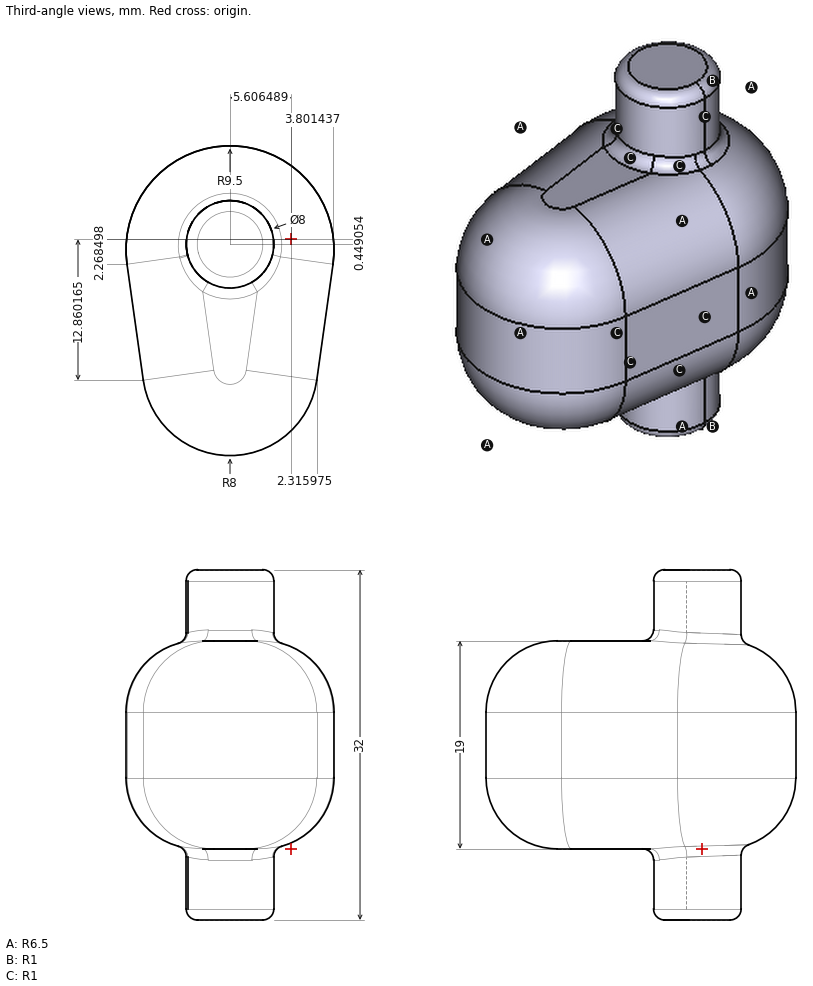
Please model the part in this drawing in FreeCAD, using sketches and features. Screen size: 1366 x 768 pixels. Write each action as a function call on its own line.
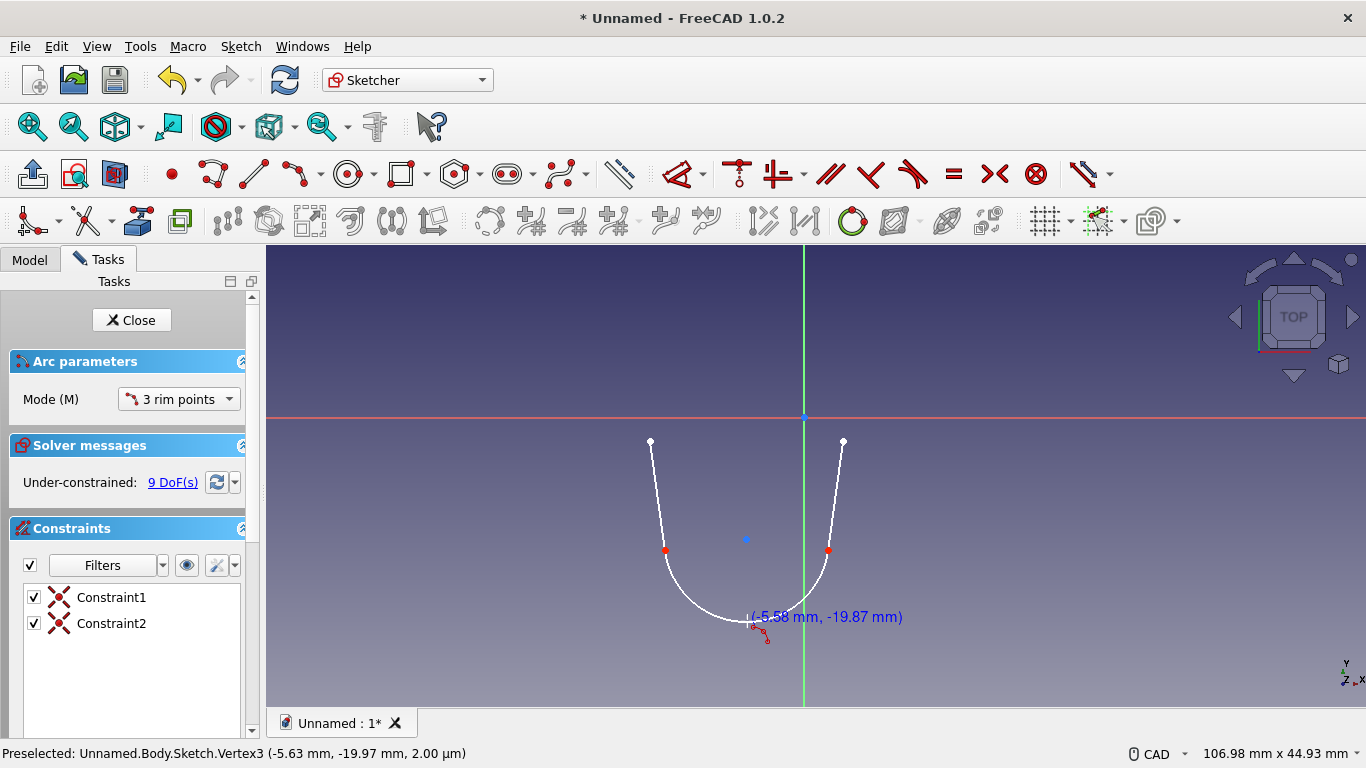
click(843, 442)
click(650, 442)
click(747, 330)
key(Escape)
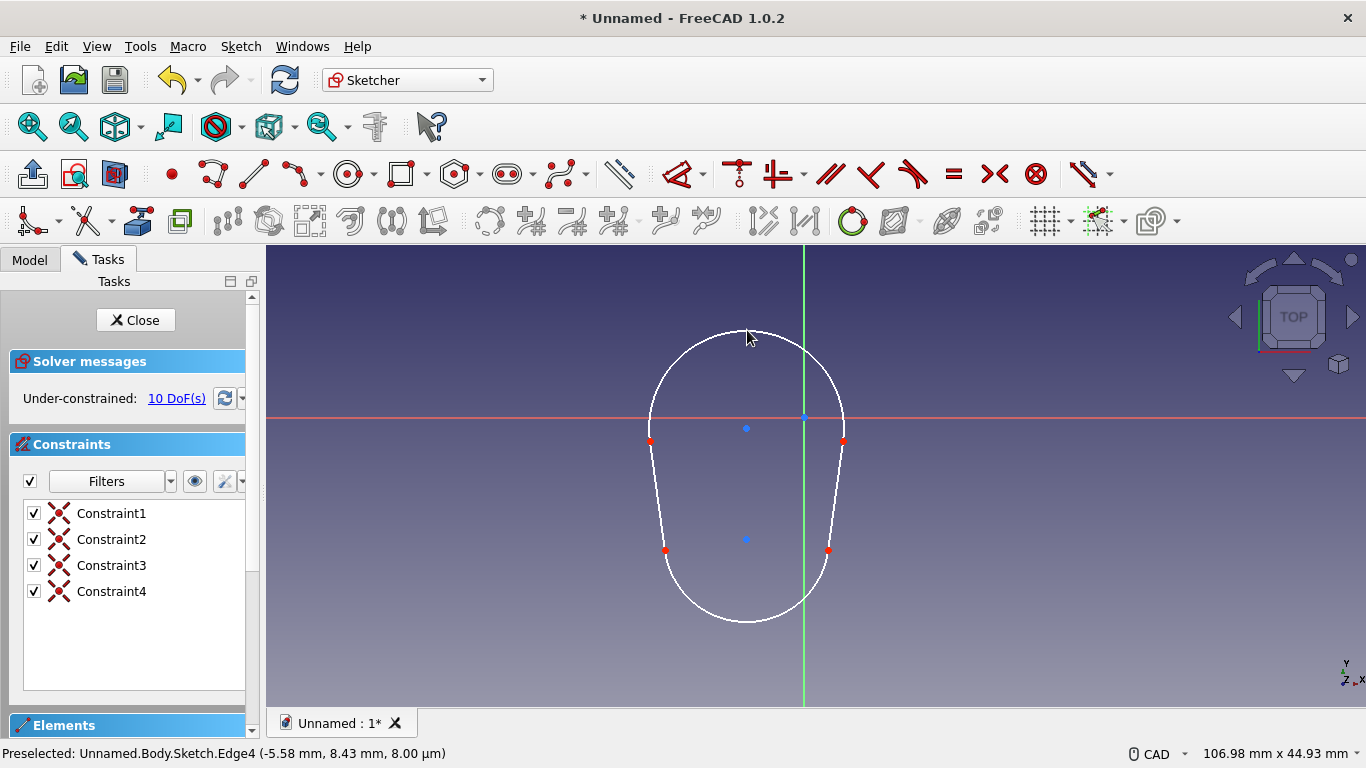
click(654, 475)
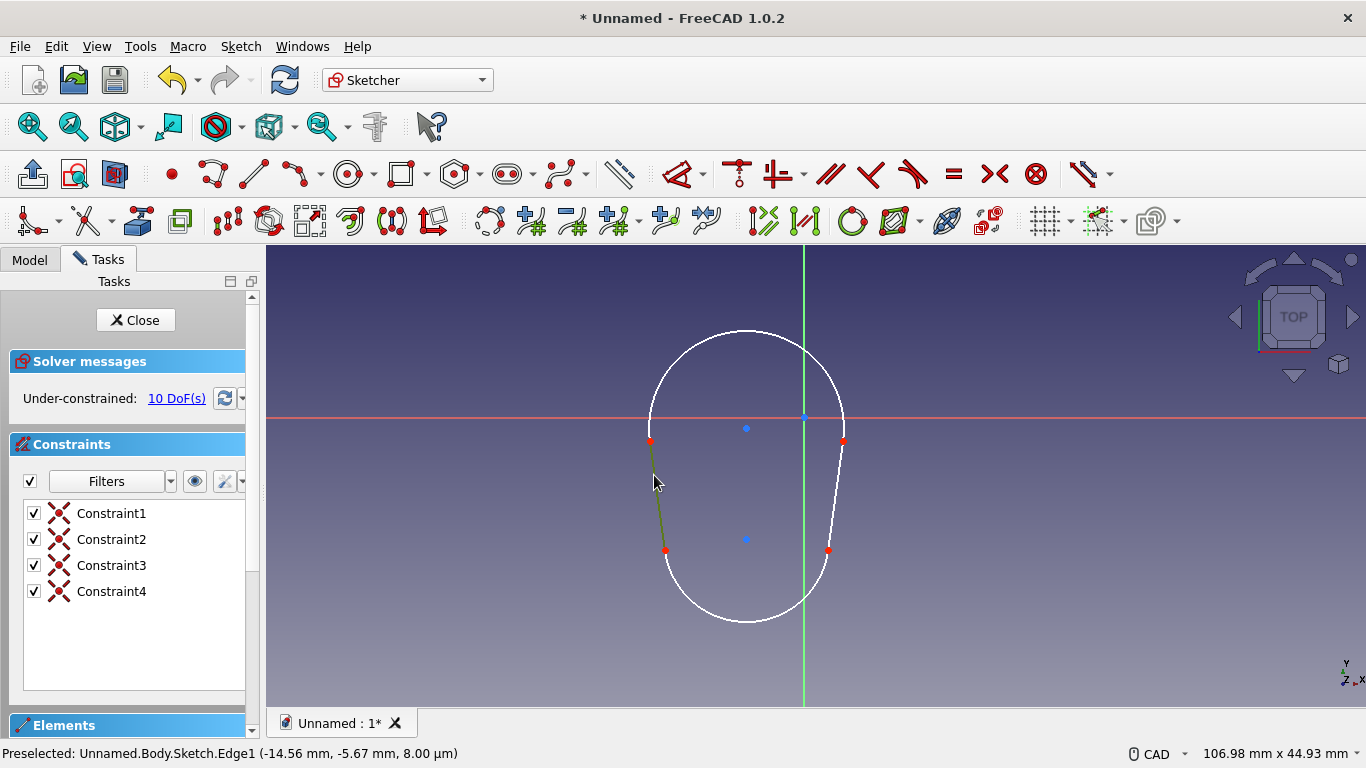
click(702, 609)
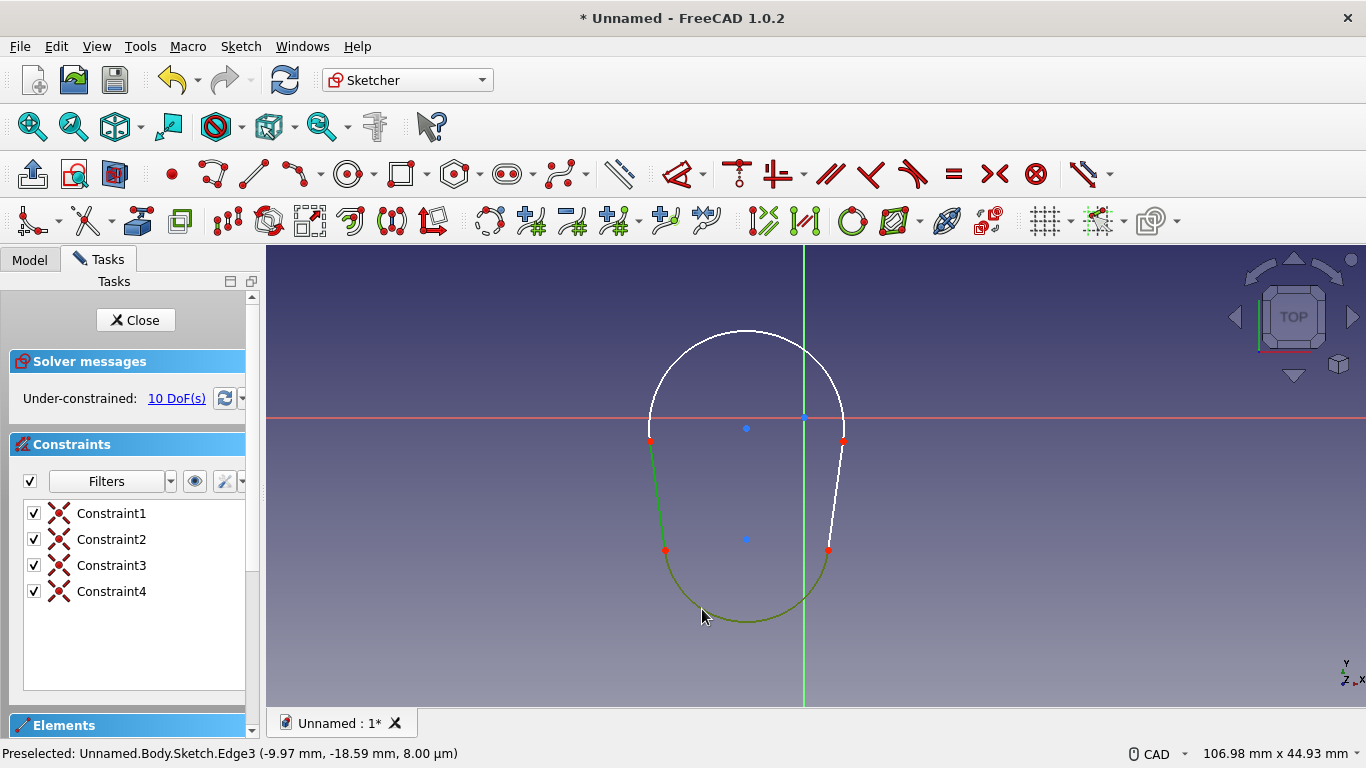
key(t)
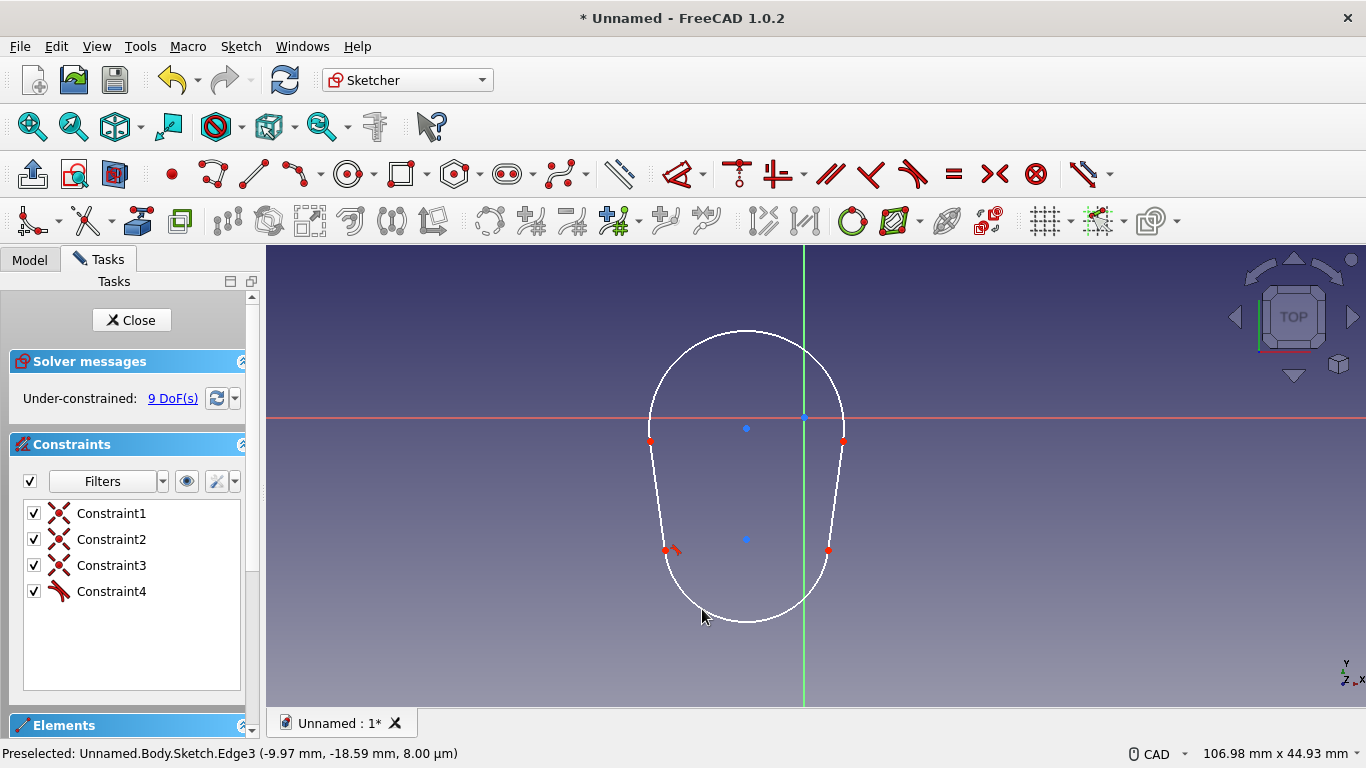
click(654, 475)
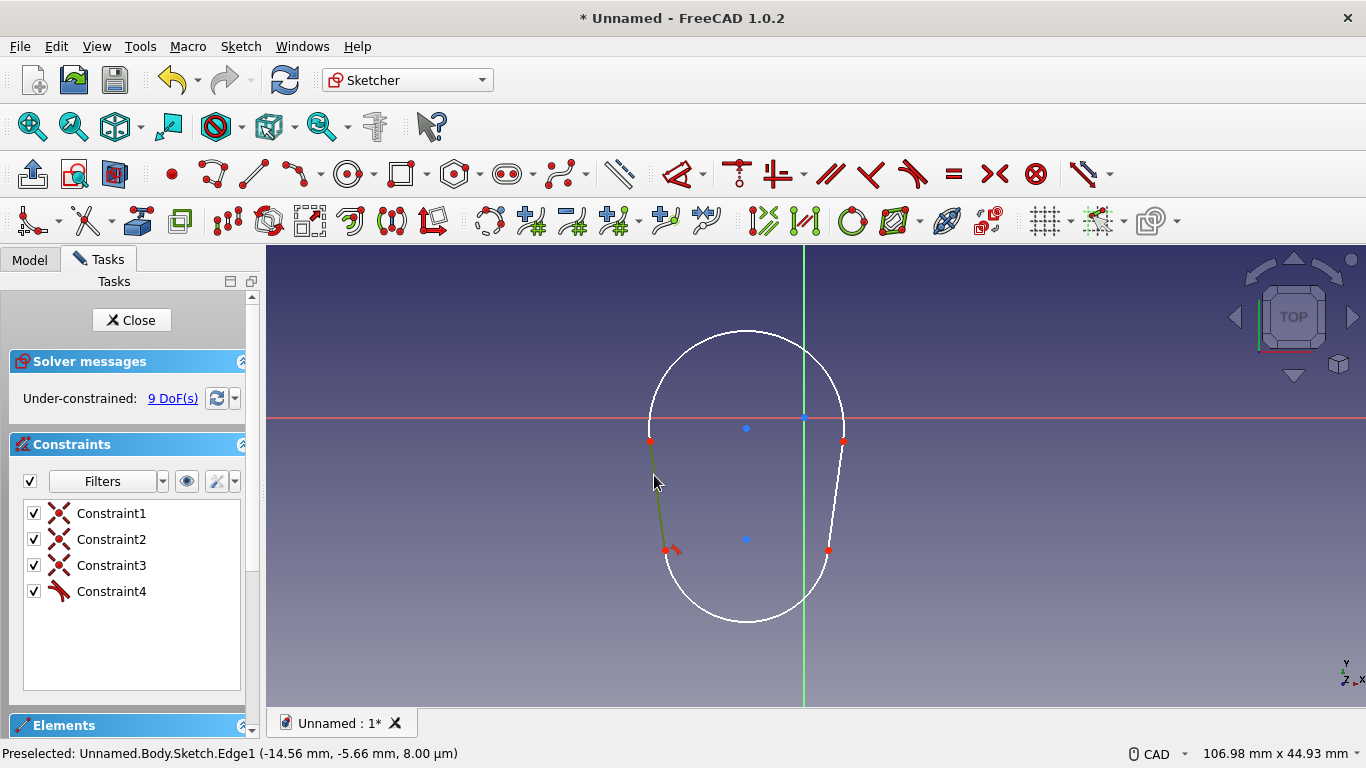
click(808, 353)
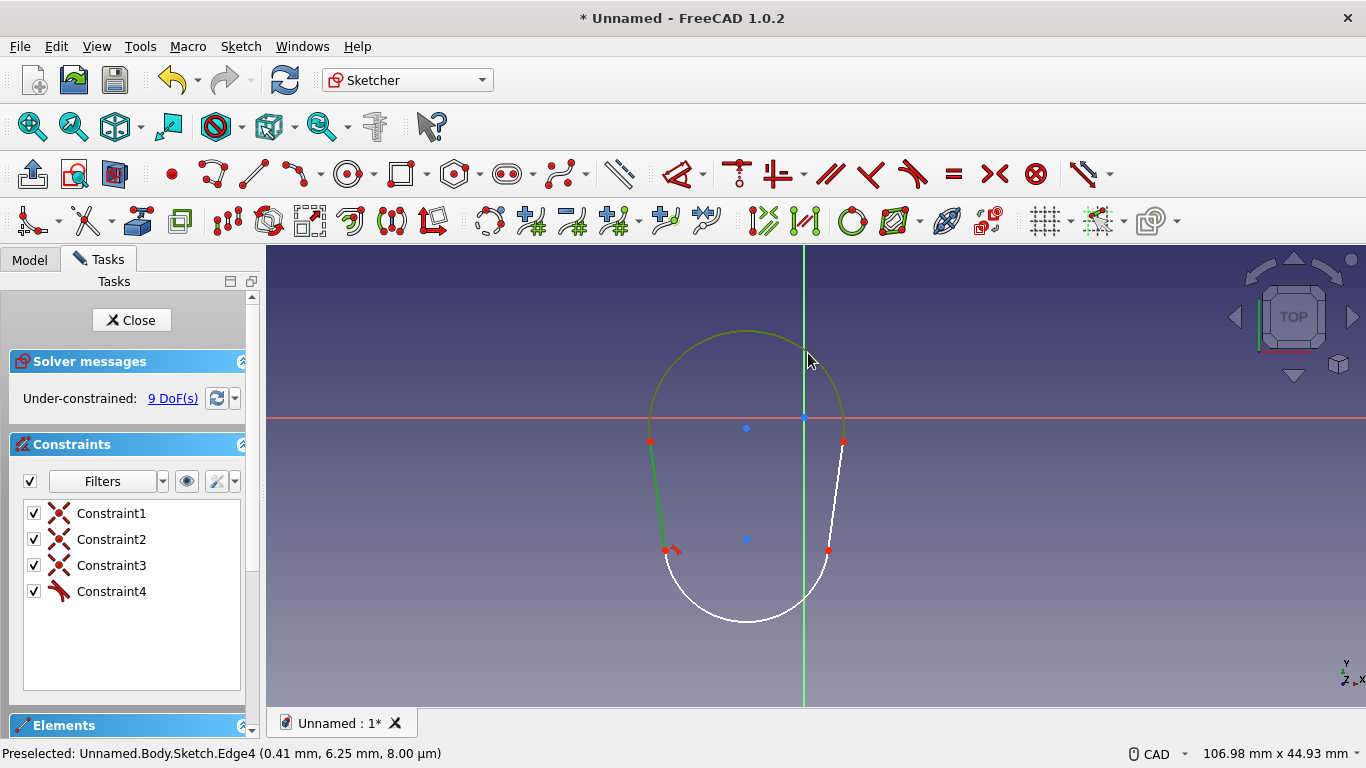
key(t)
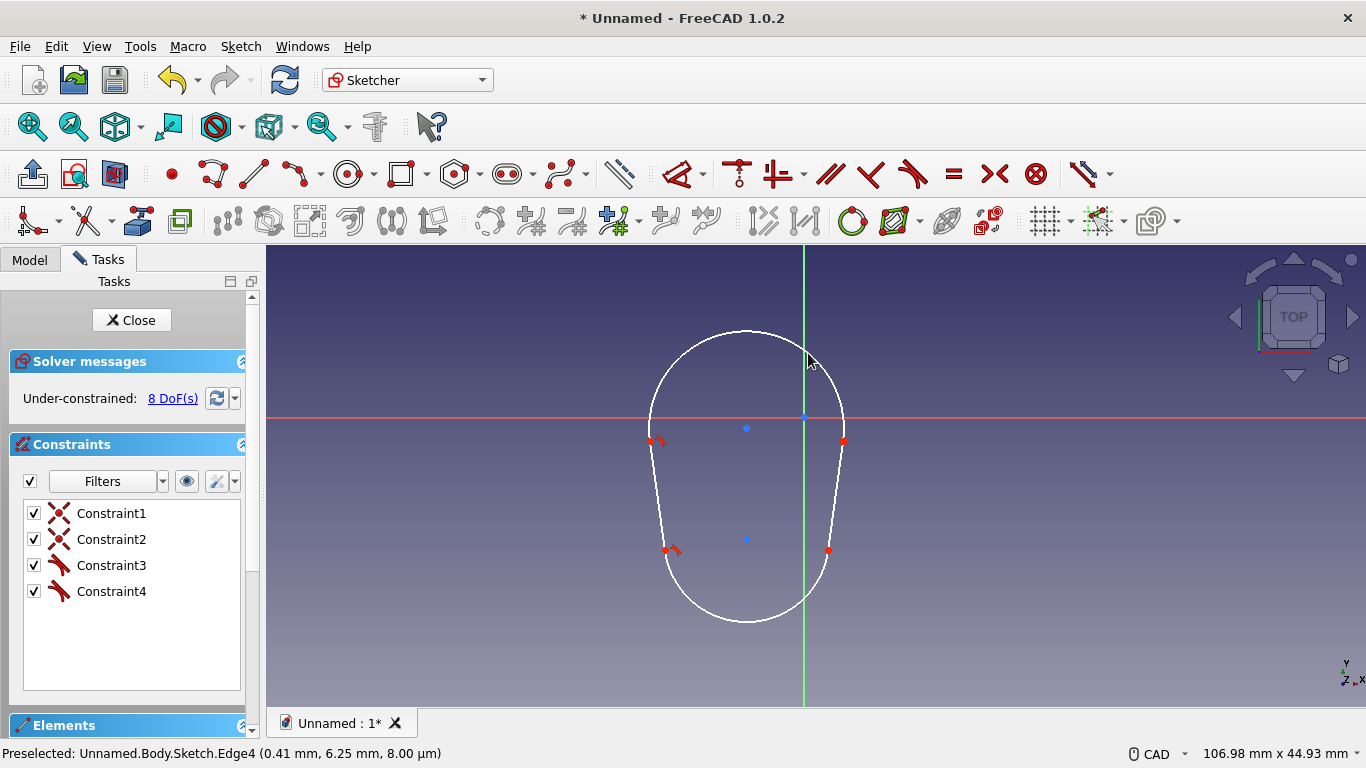
click(832, 518)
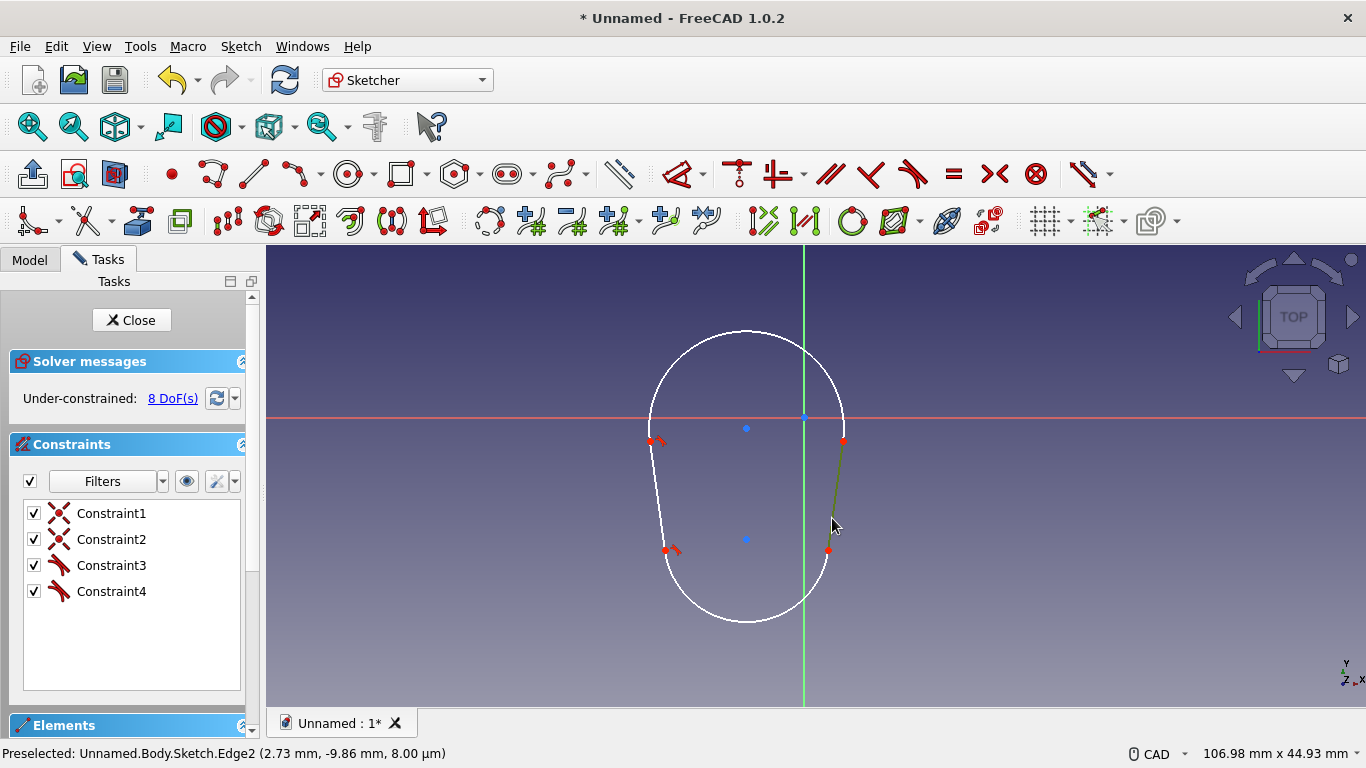
click(702, 609)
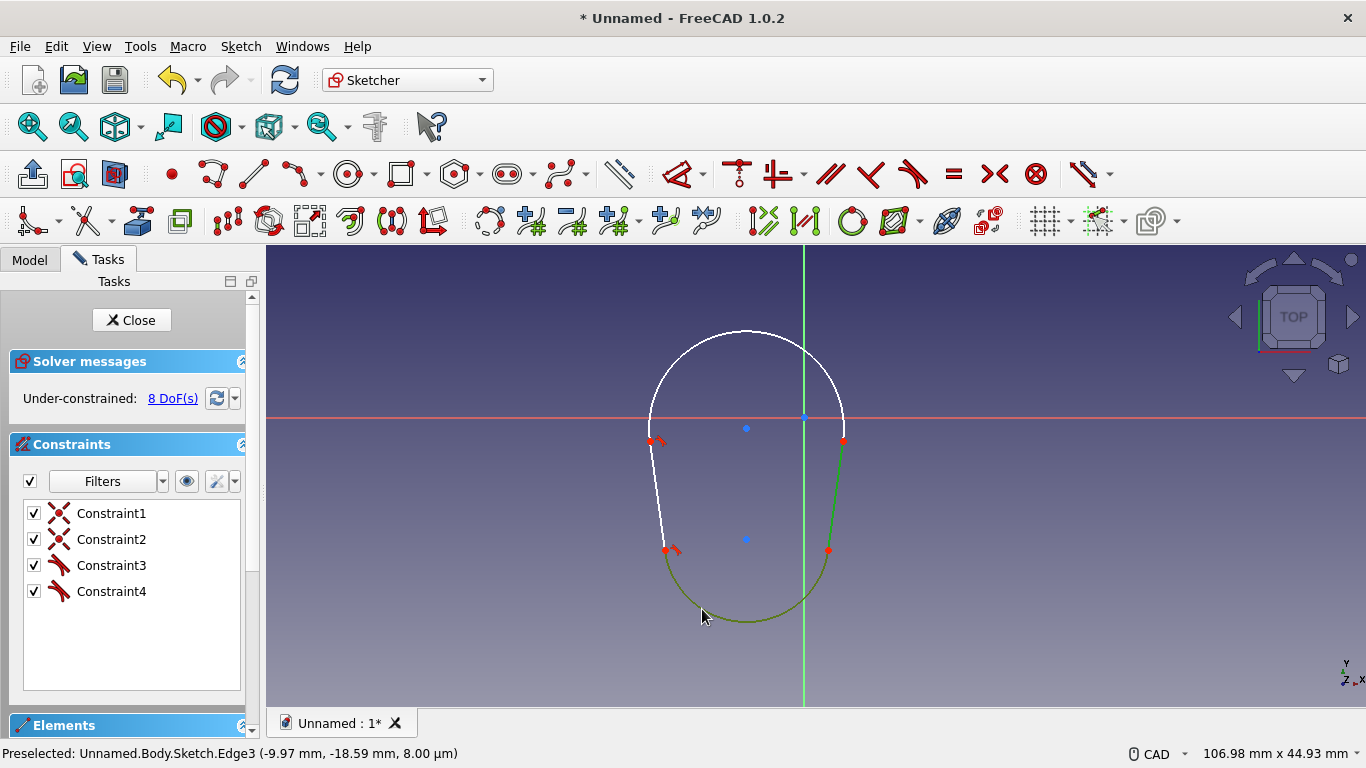
click(913, 174)